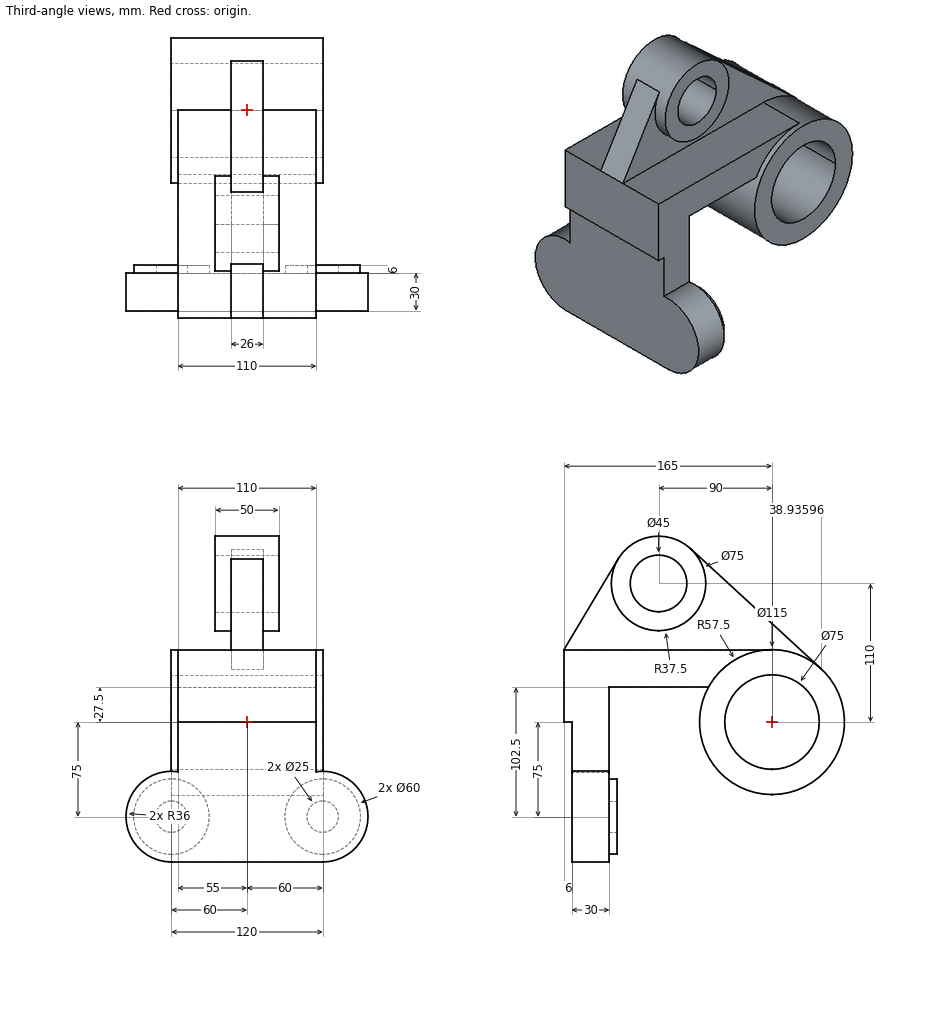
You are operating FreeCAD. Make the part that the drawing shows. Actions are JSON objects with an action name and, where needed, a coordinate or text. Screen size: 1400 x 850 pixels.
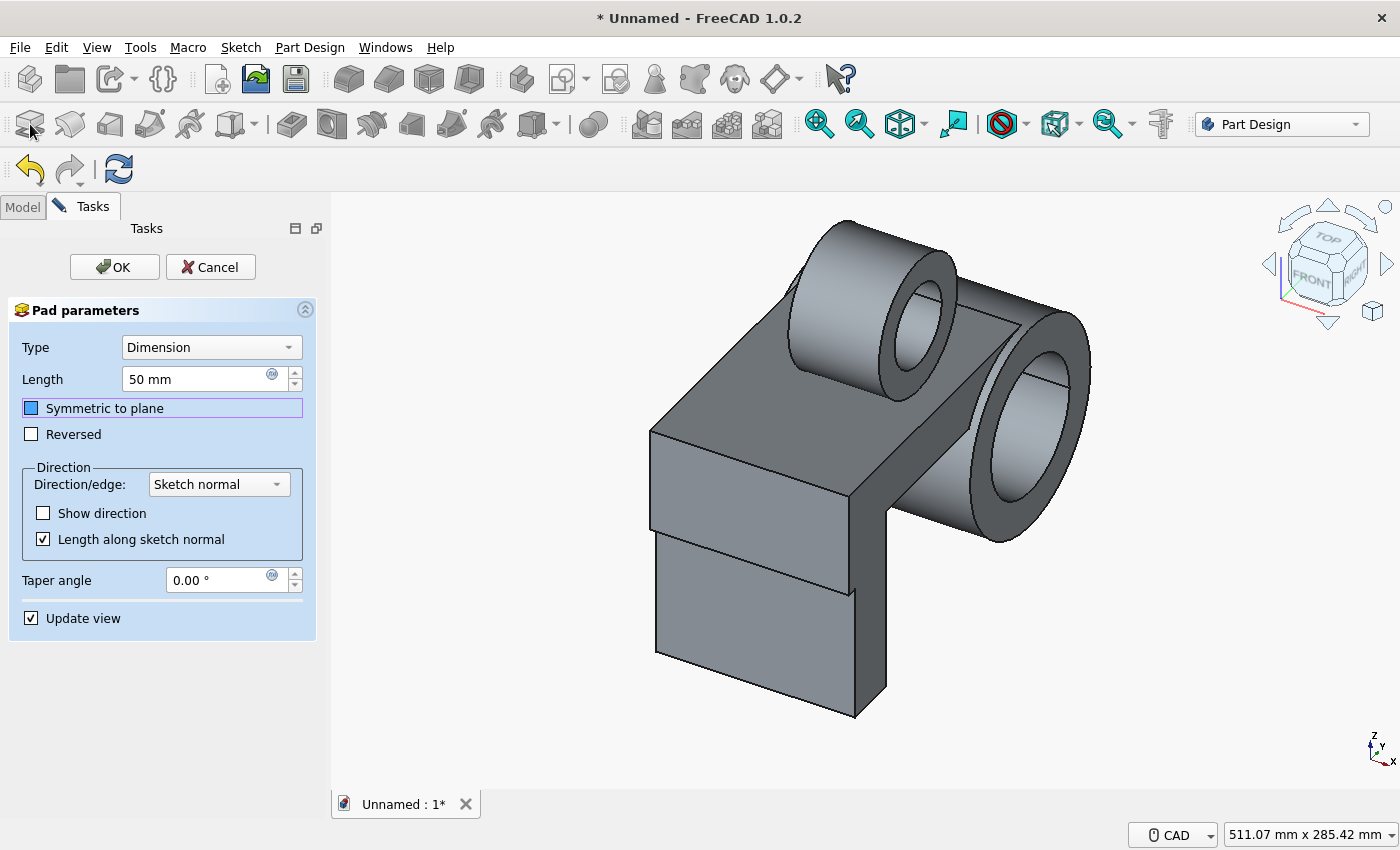
{"action": "left_click", "coordinate": [30, 408]}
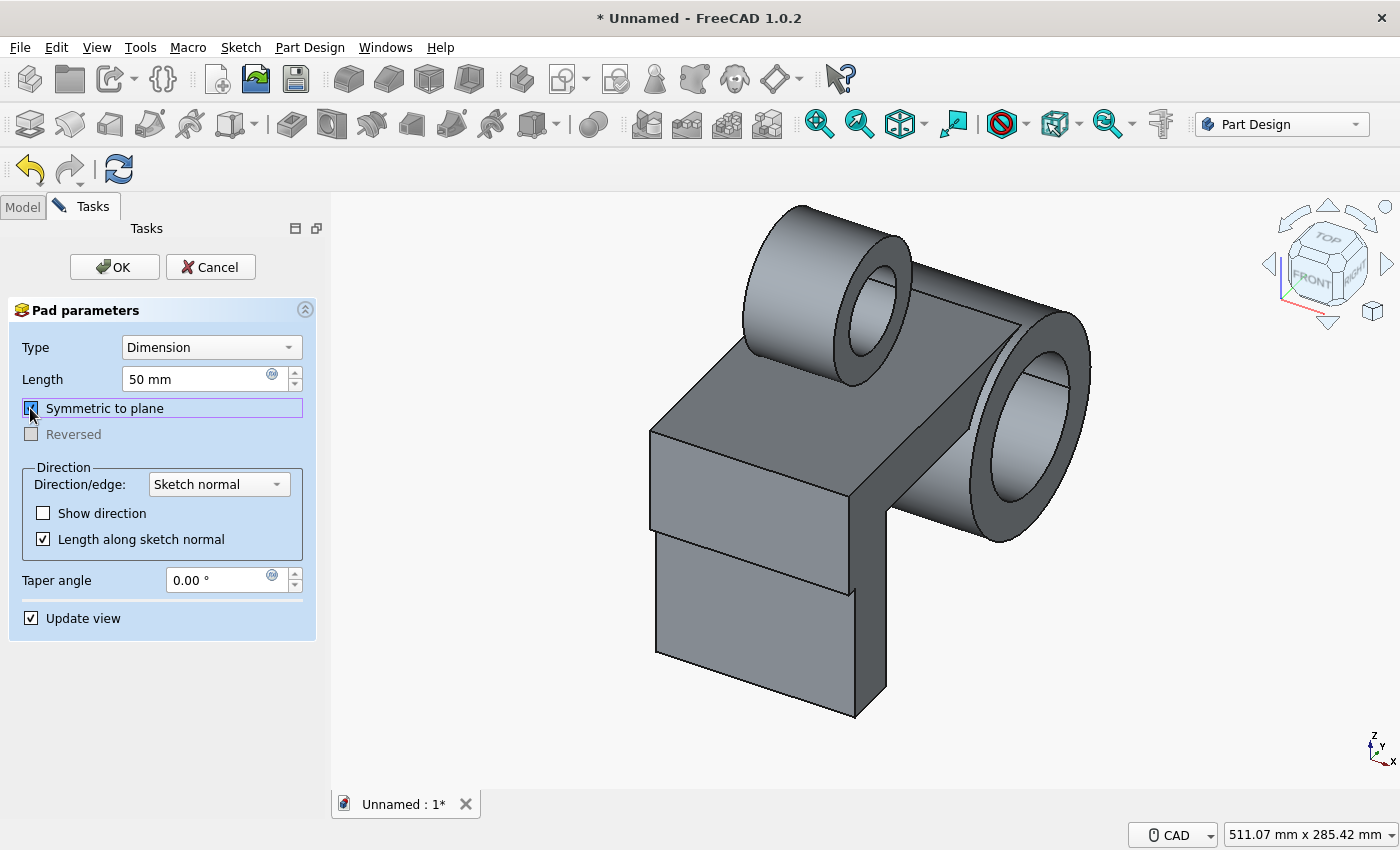
{"action": "left_click", "coordinate": [115, 267]}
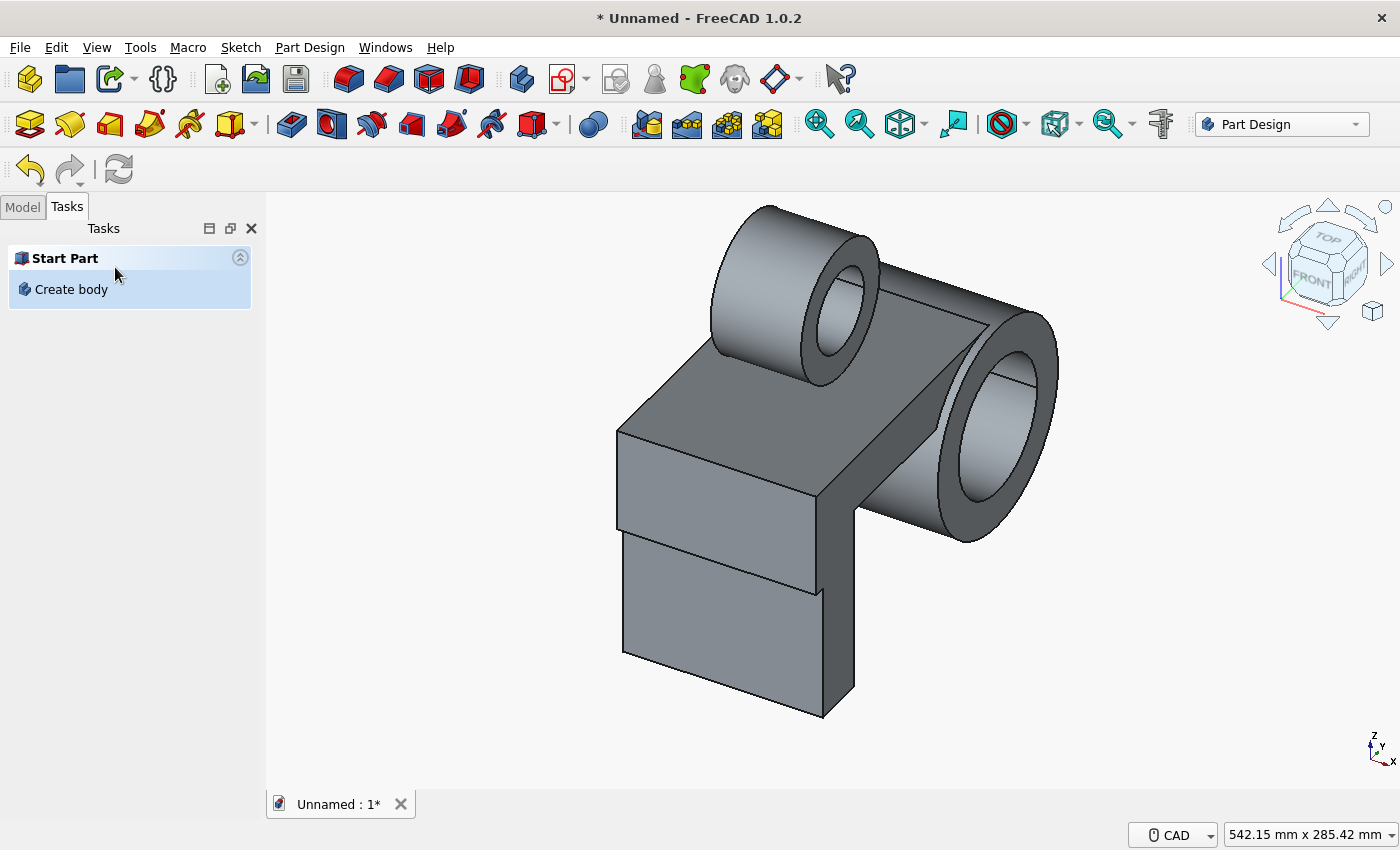
{"action": "key", "text": "v f"}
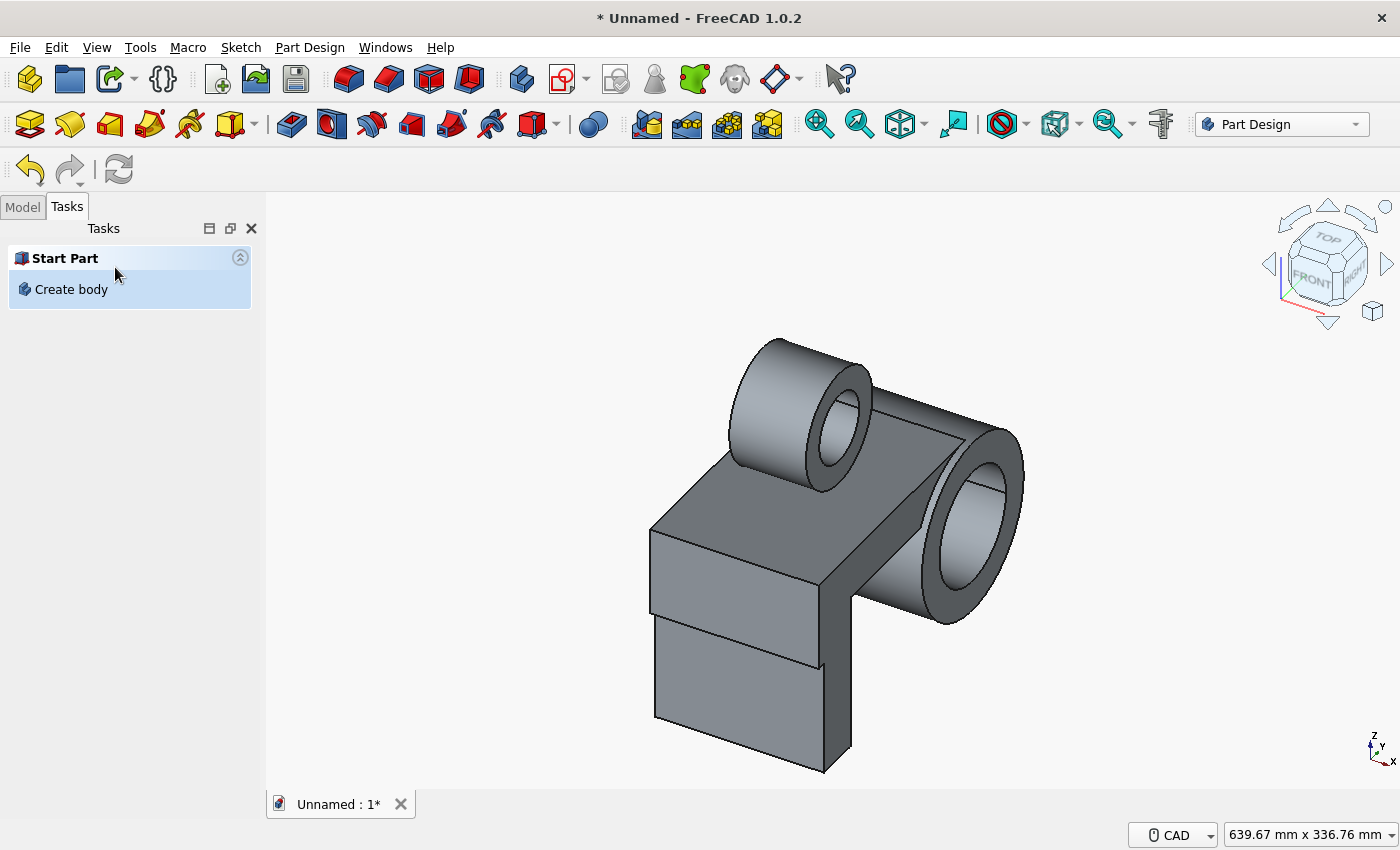
{"action": "left_click", "coordinate": [23, 206]}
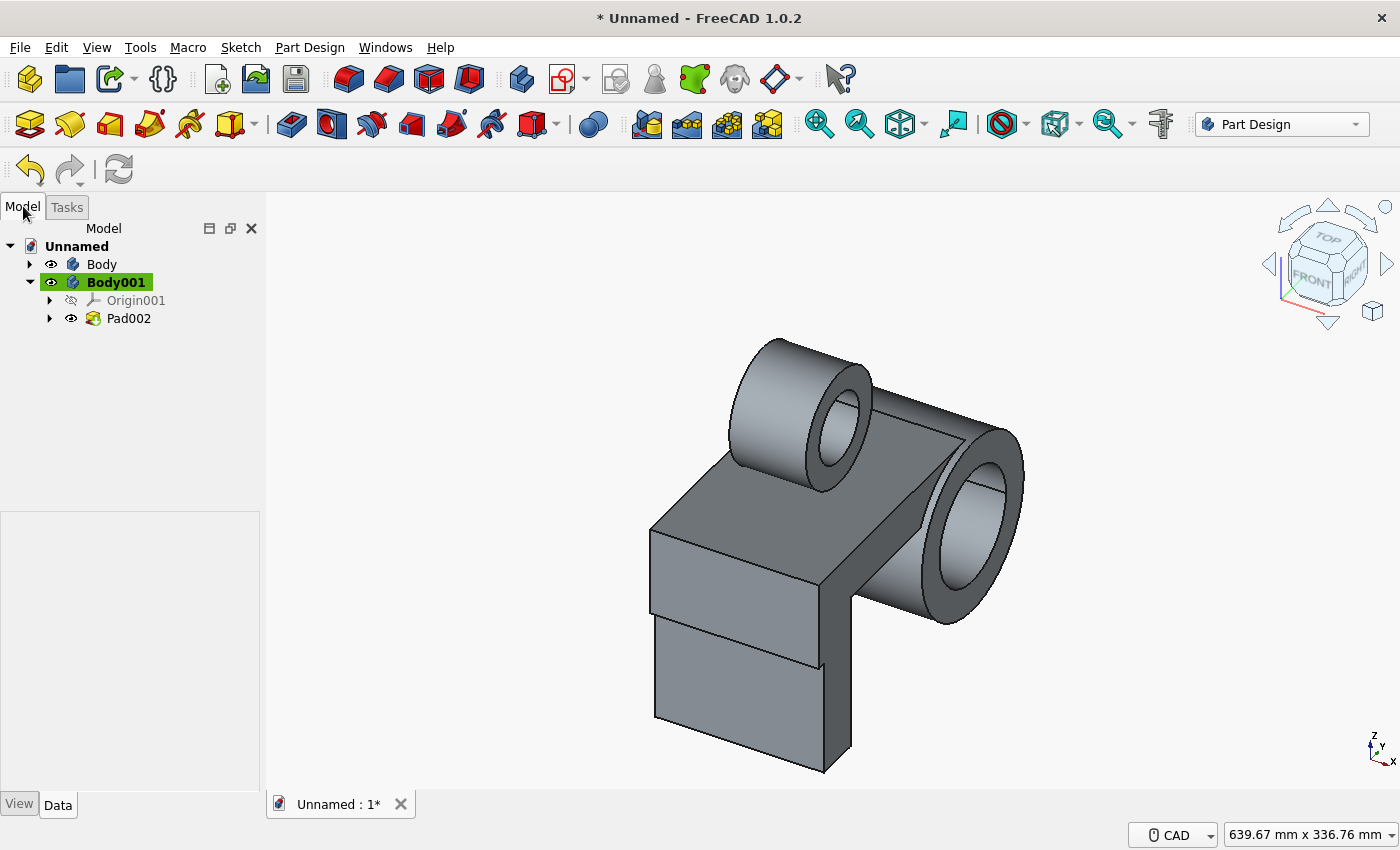
{"action": "double_click", "coordinate": [96, 264]}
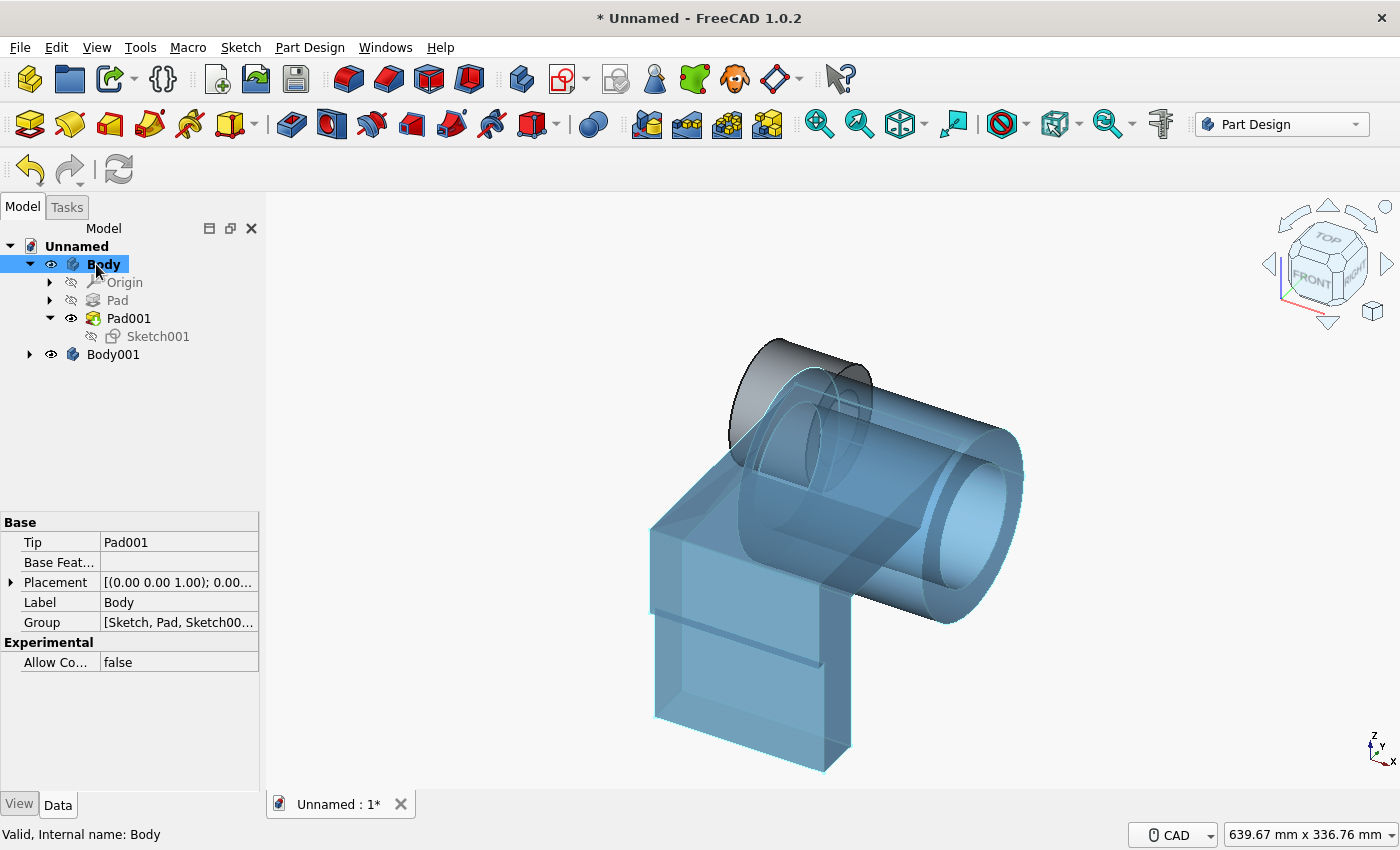
{"action": "left_click", "coordinate": [96, 264]}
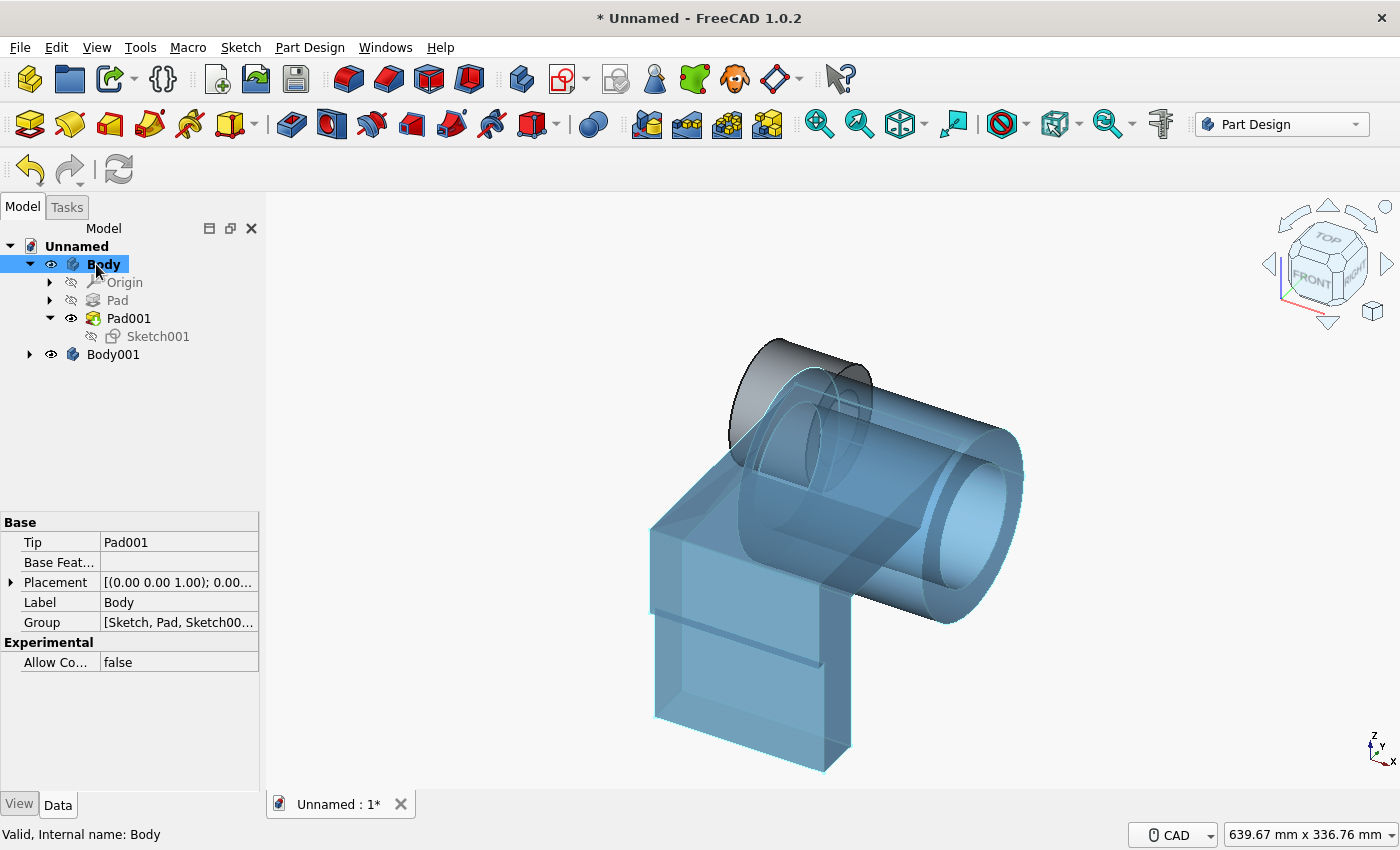
{"action": "left_click", "coordinate": [146, 662]}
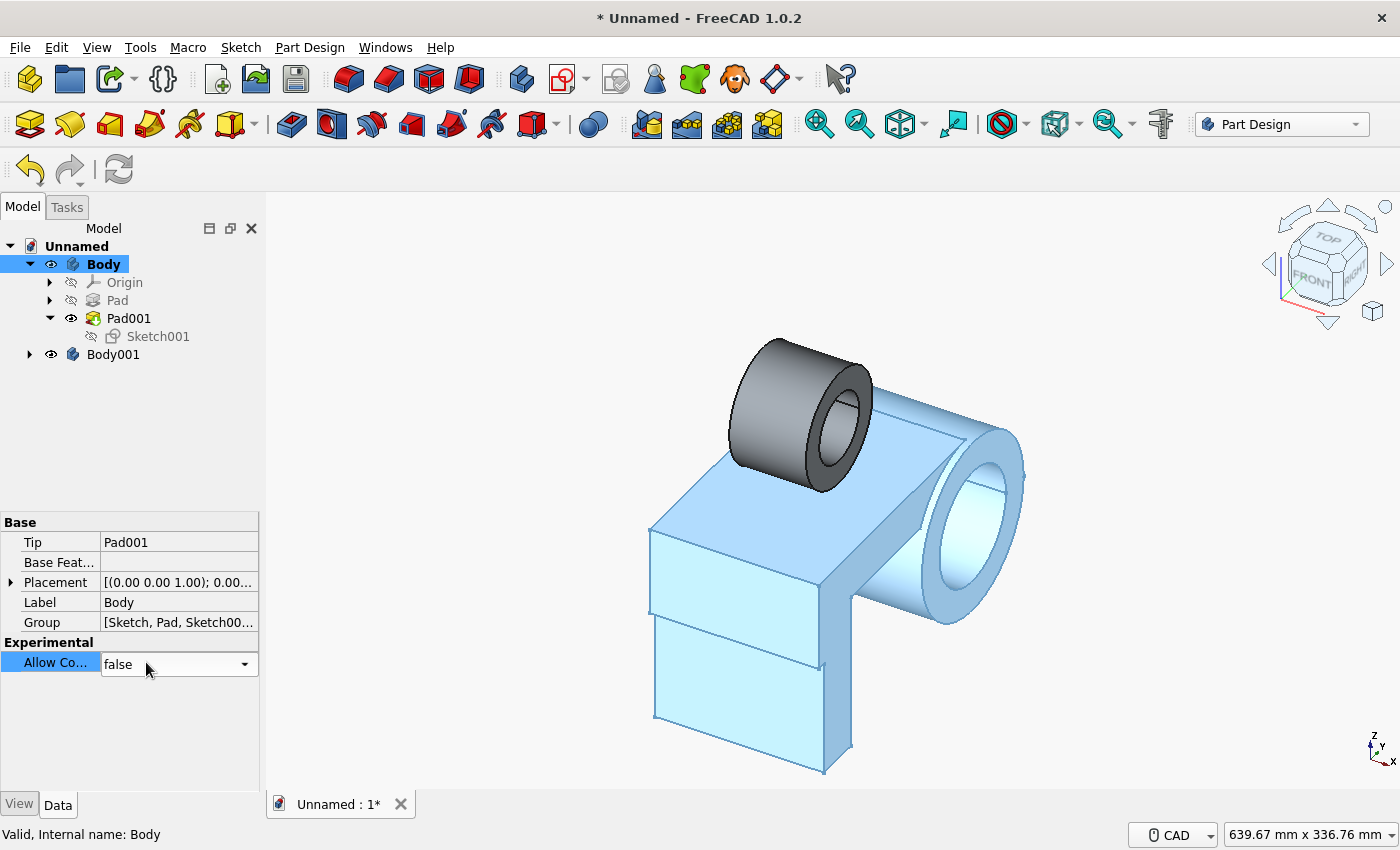
{"action": "left_click", "coordinate": [146, 662]}